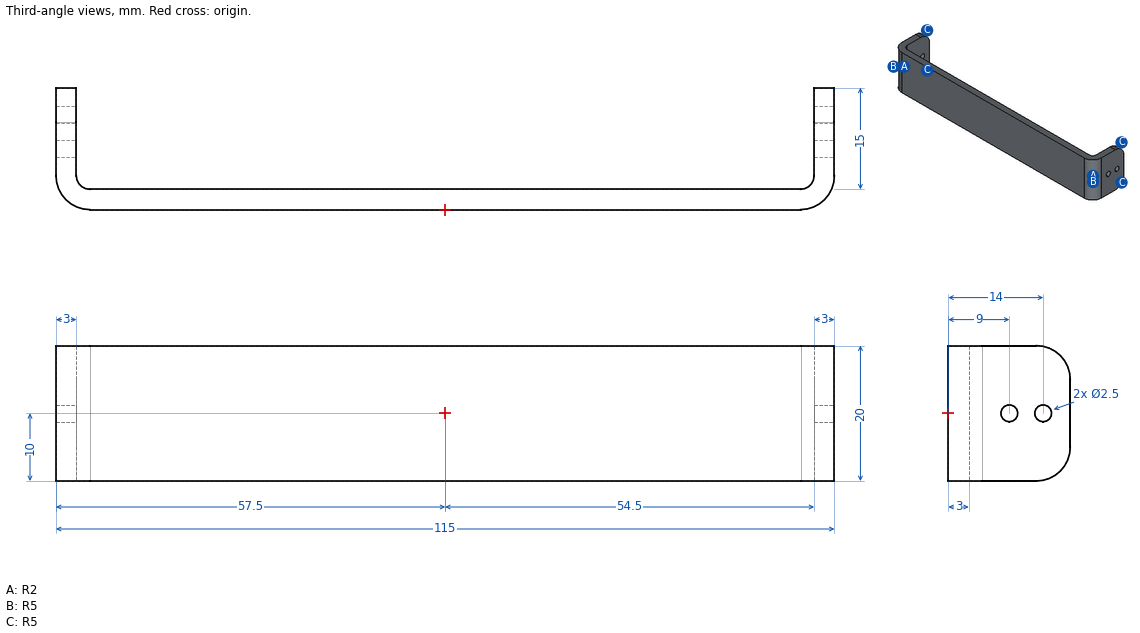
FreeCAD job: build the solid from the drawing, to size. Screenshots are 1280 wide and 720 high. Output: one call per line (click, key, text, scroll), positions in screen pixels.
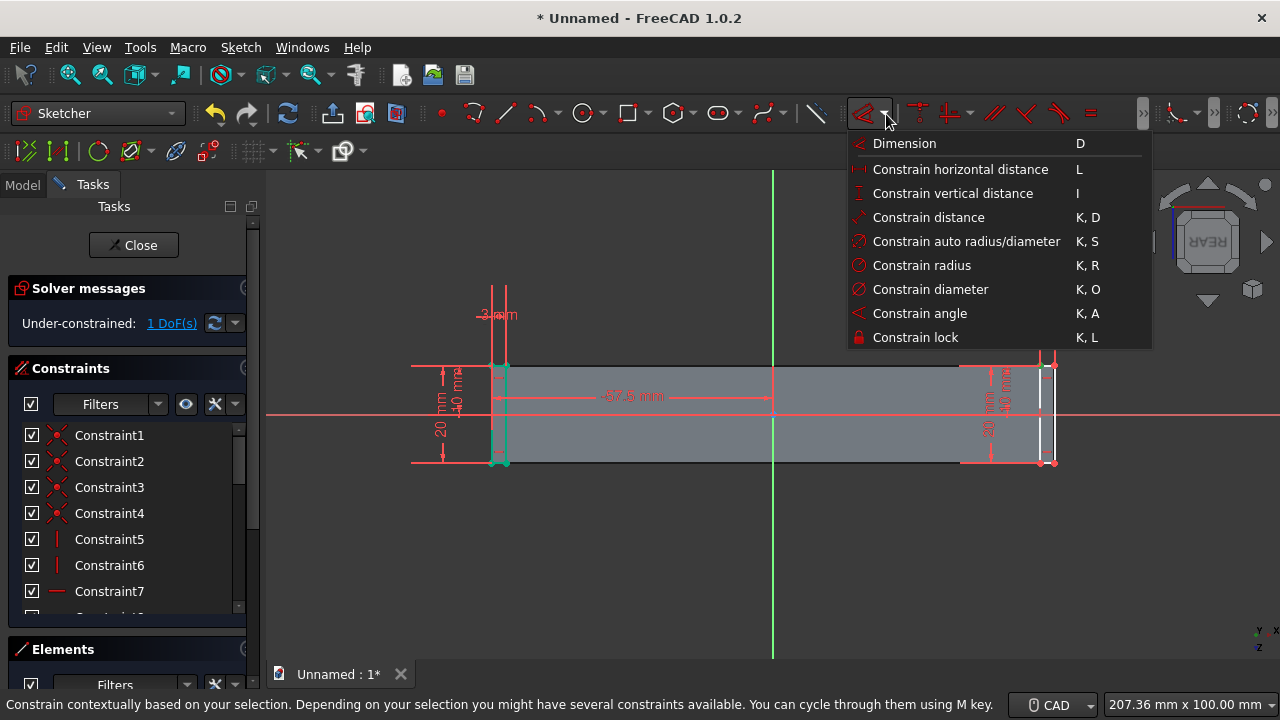
click(1000, 169)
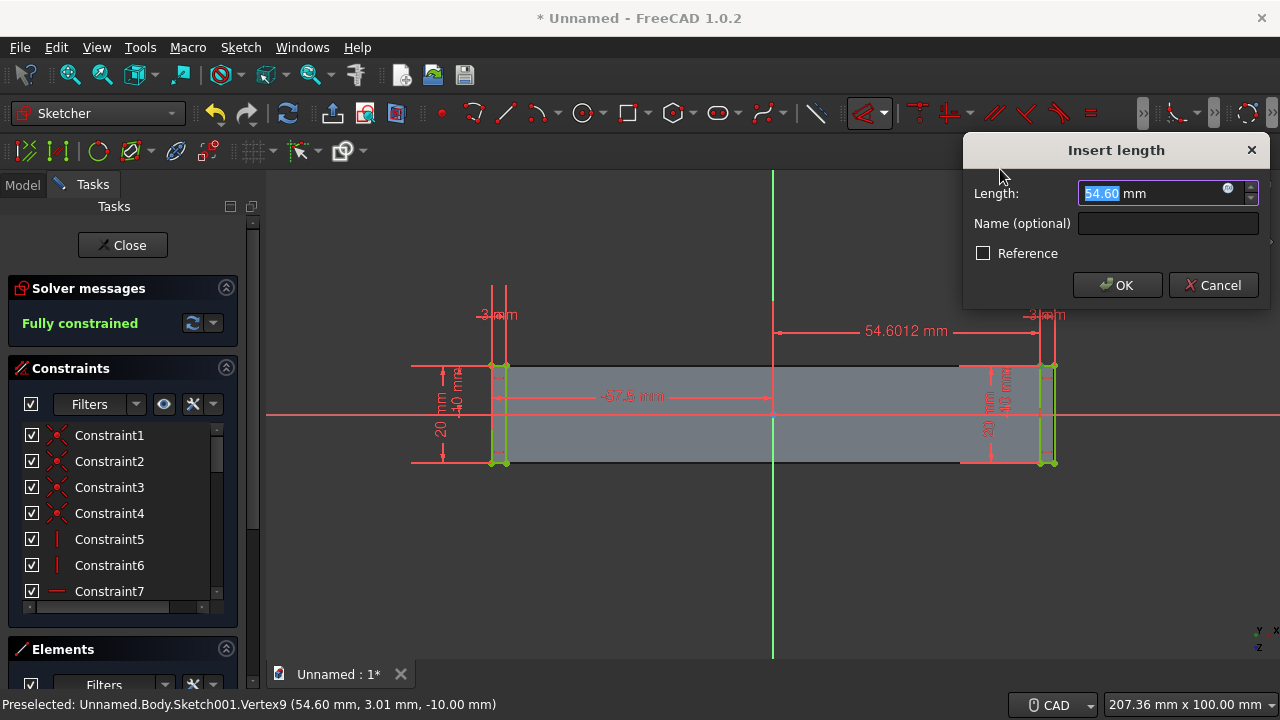
text(54.5)
key(Return)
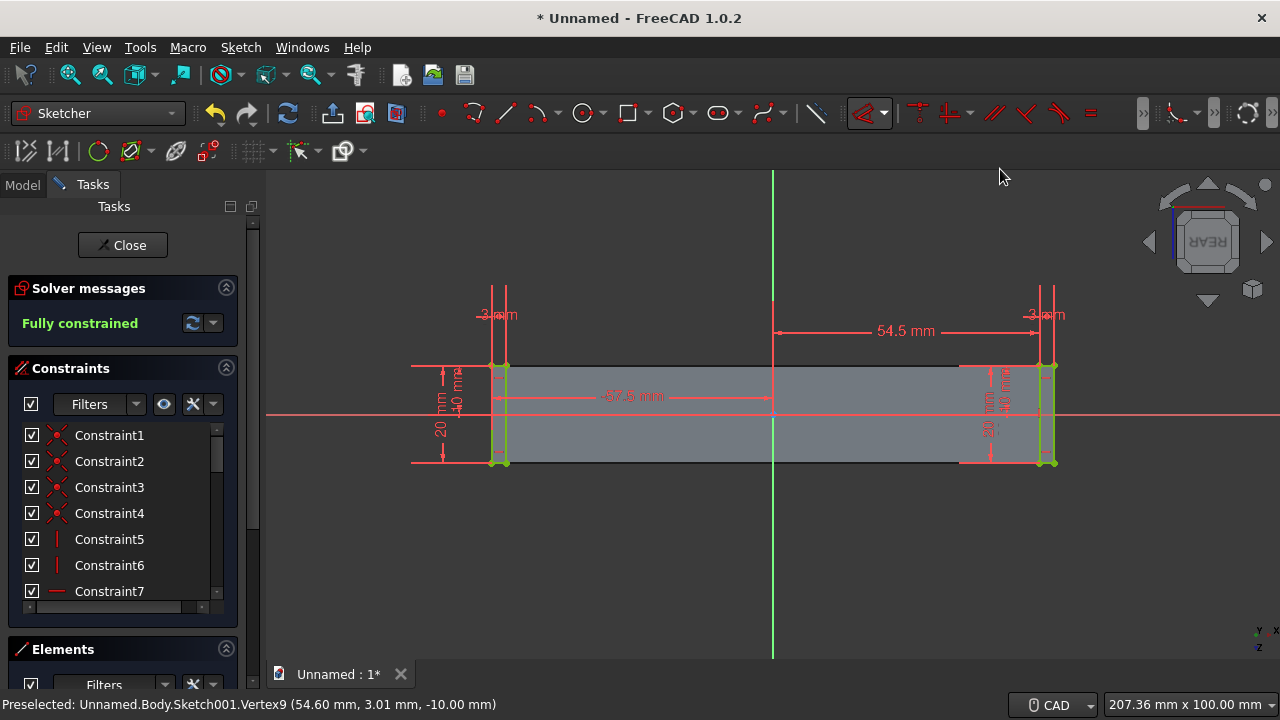
click(123, 245)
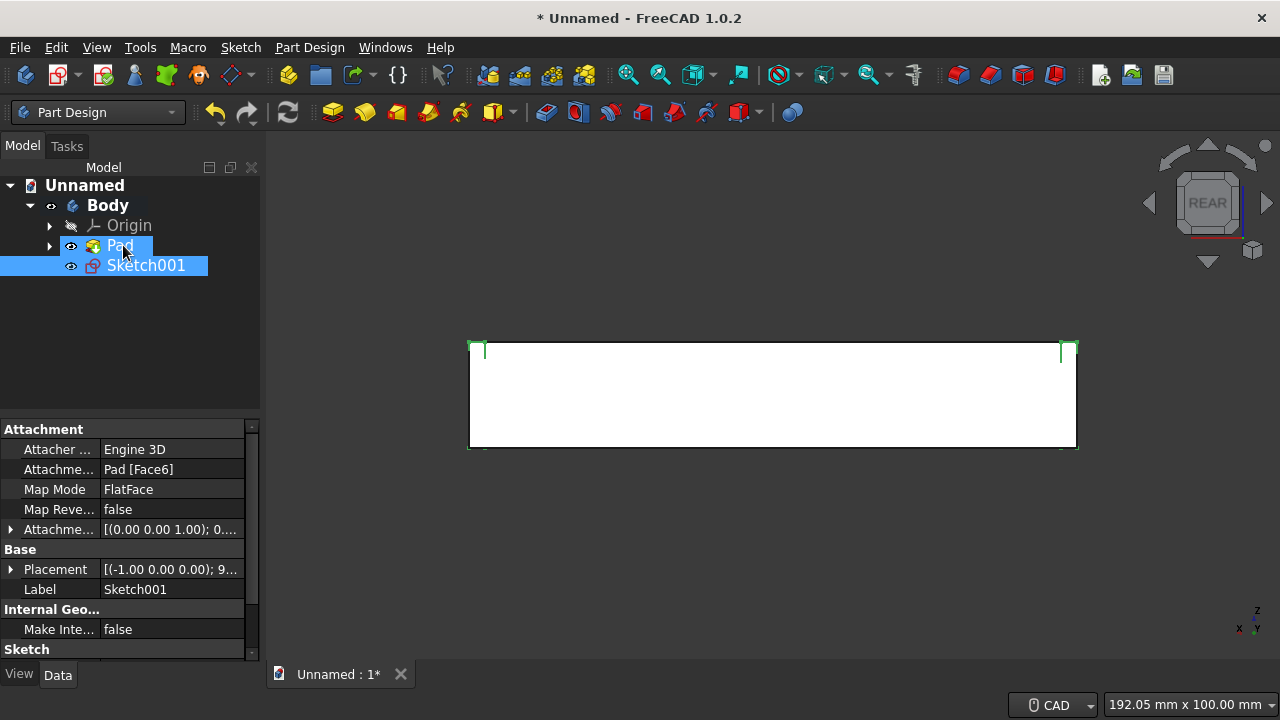
click(334, 112)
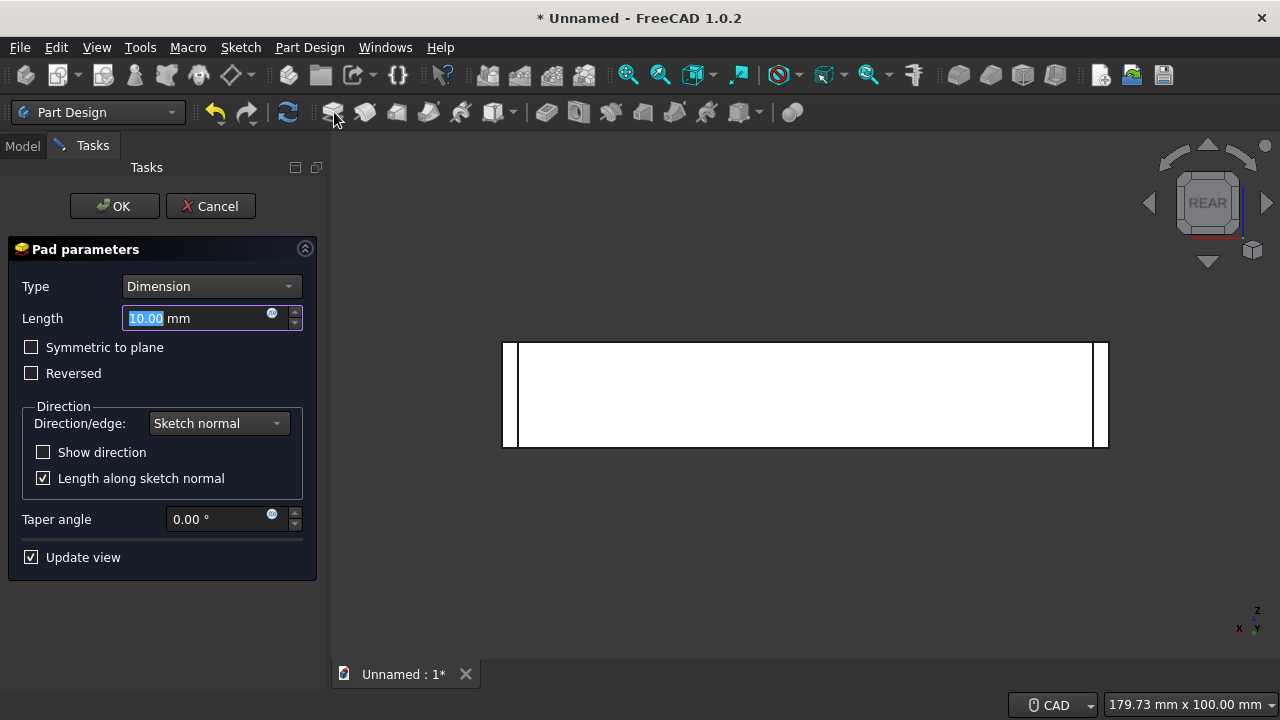
text(15)
key(Tab)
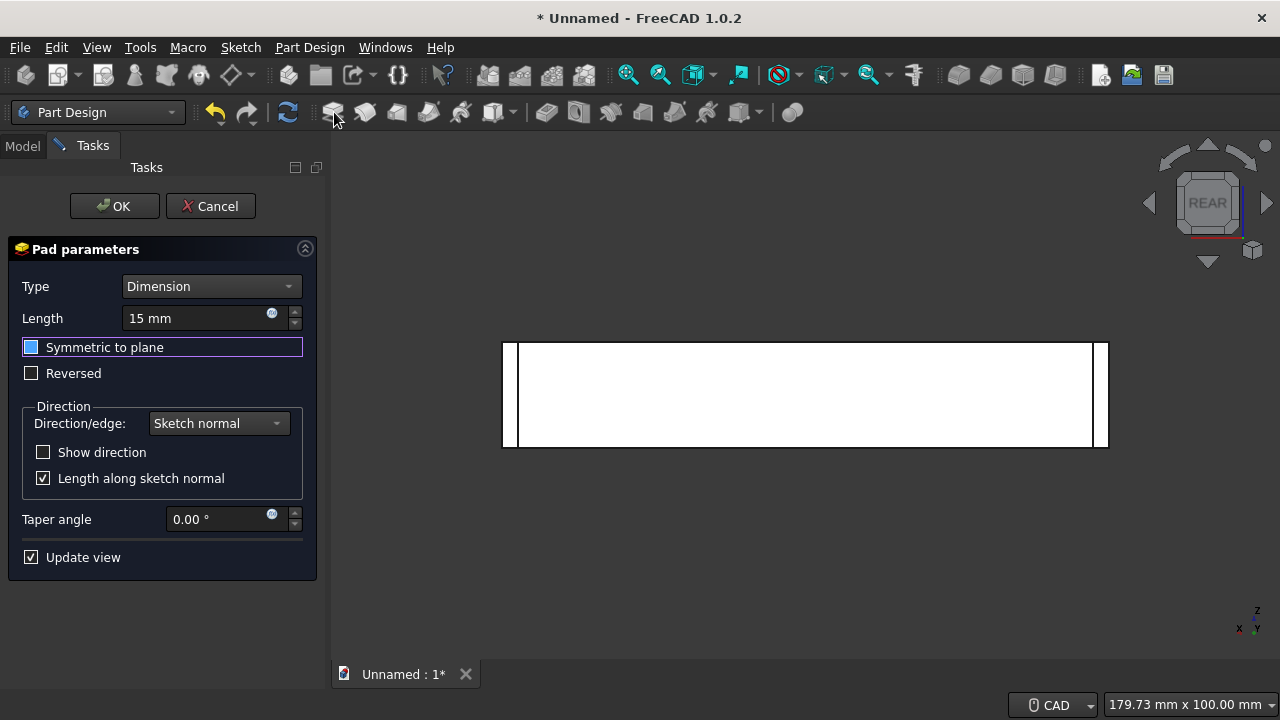
click(115, 206)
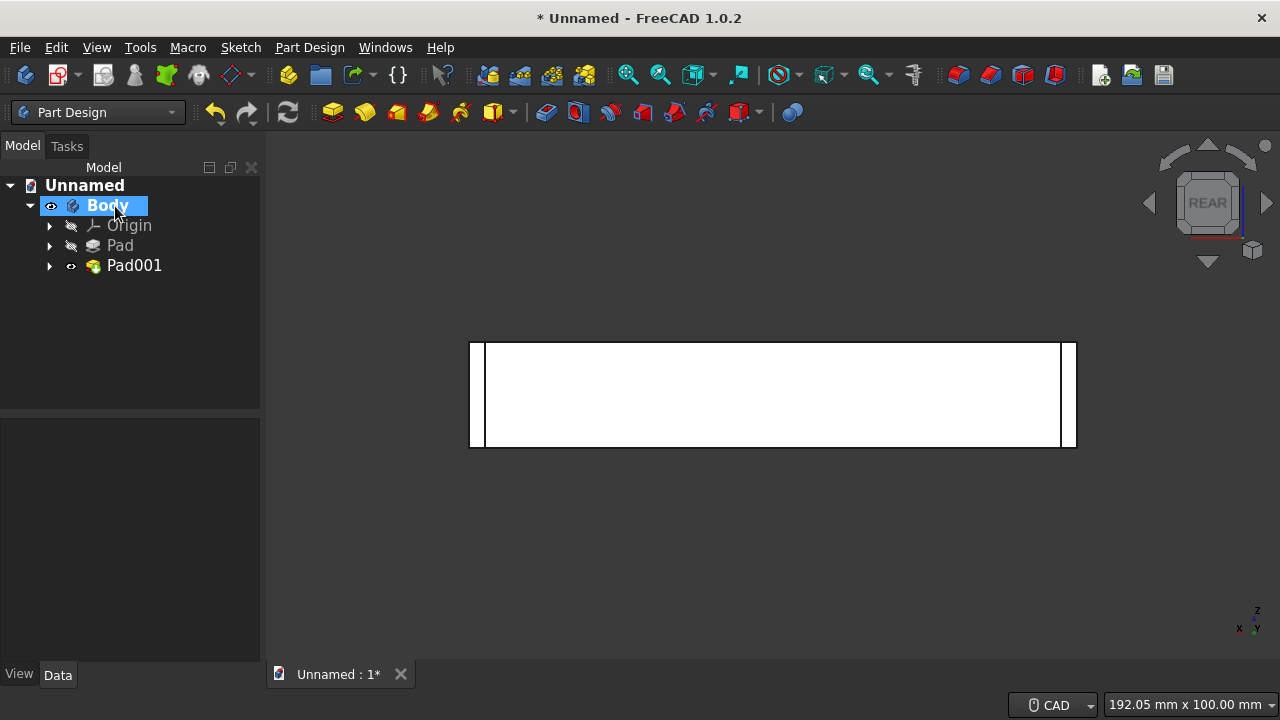
key(0)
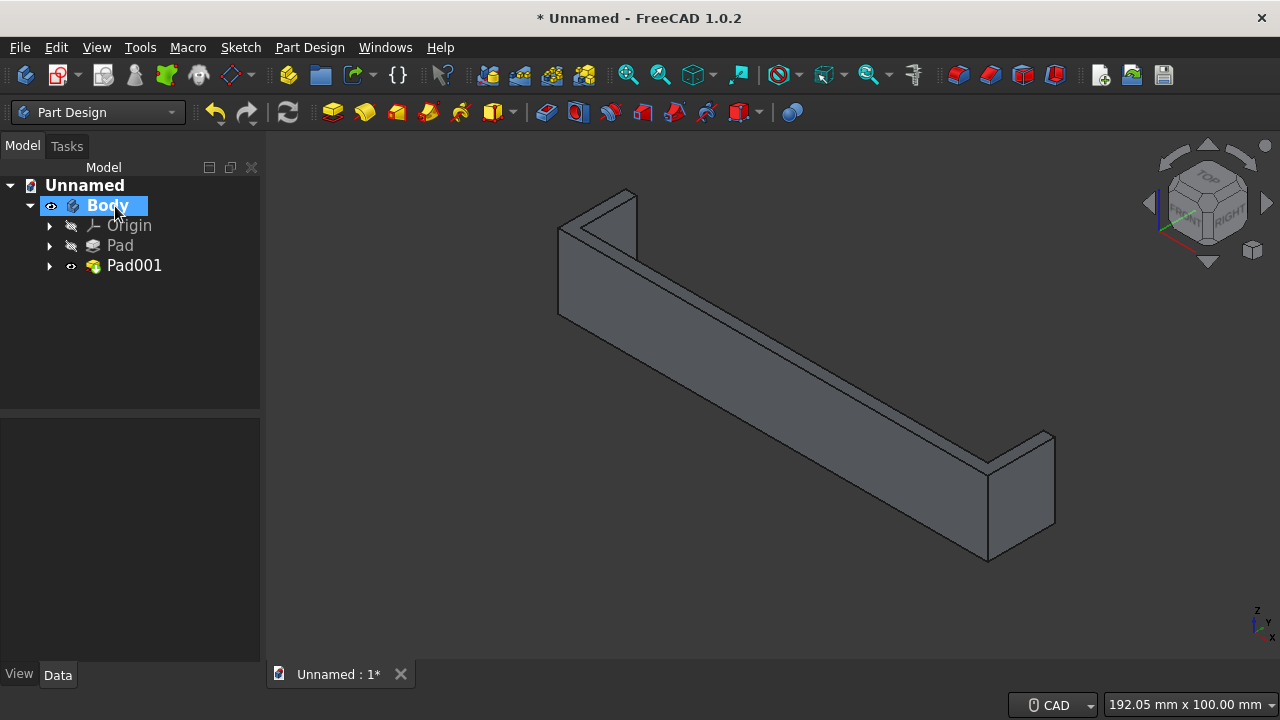
key(2)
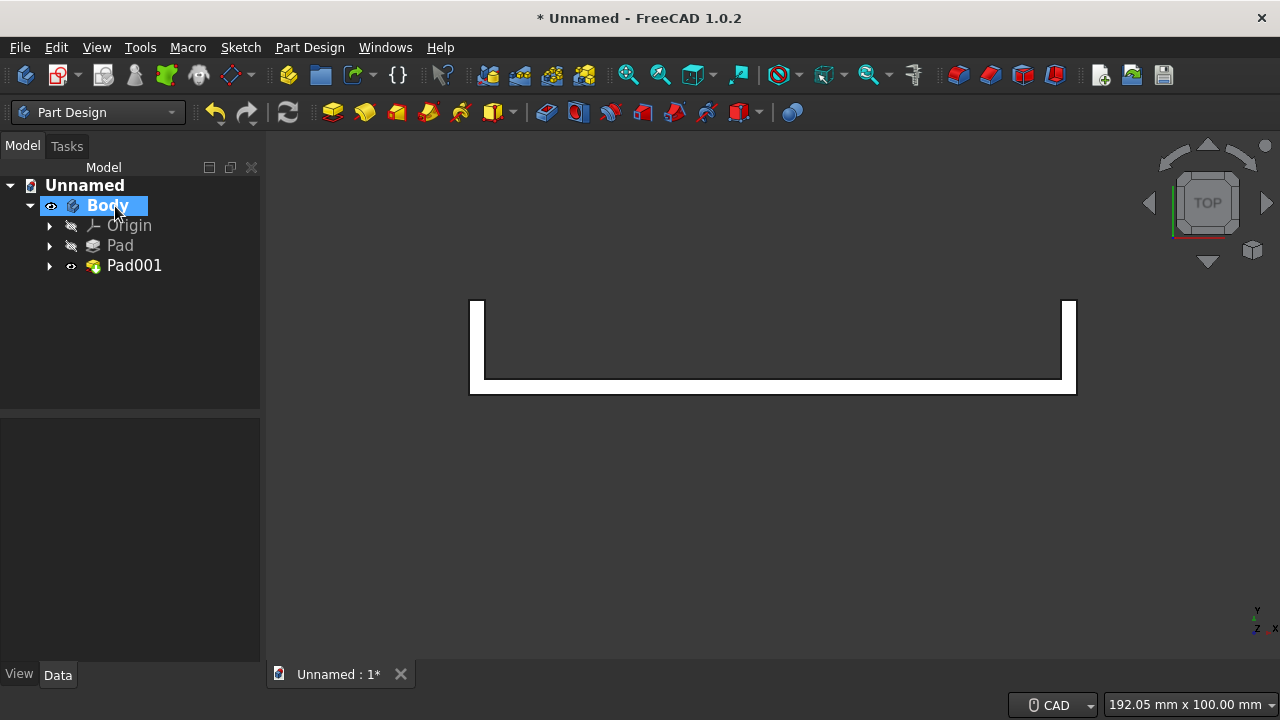
key(1)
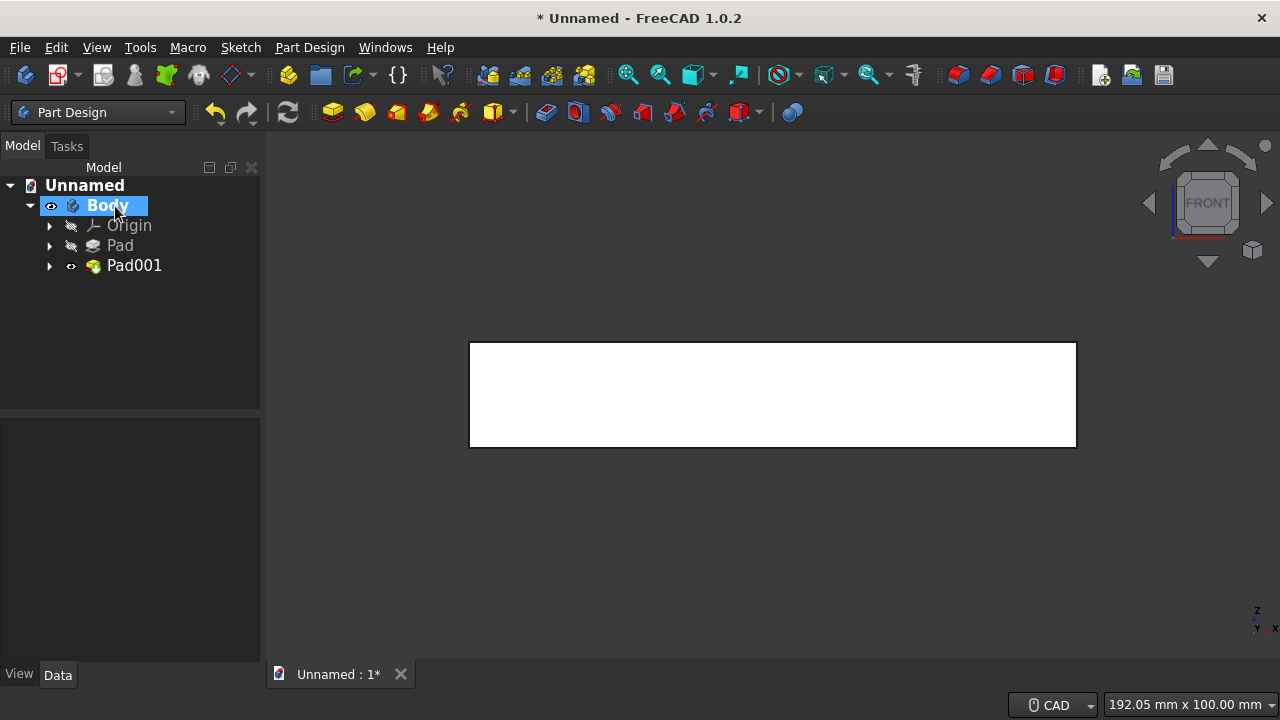
key(3)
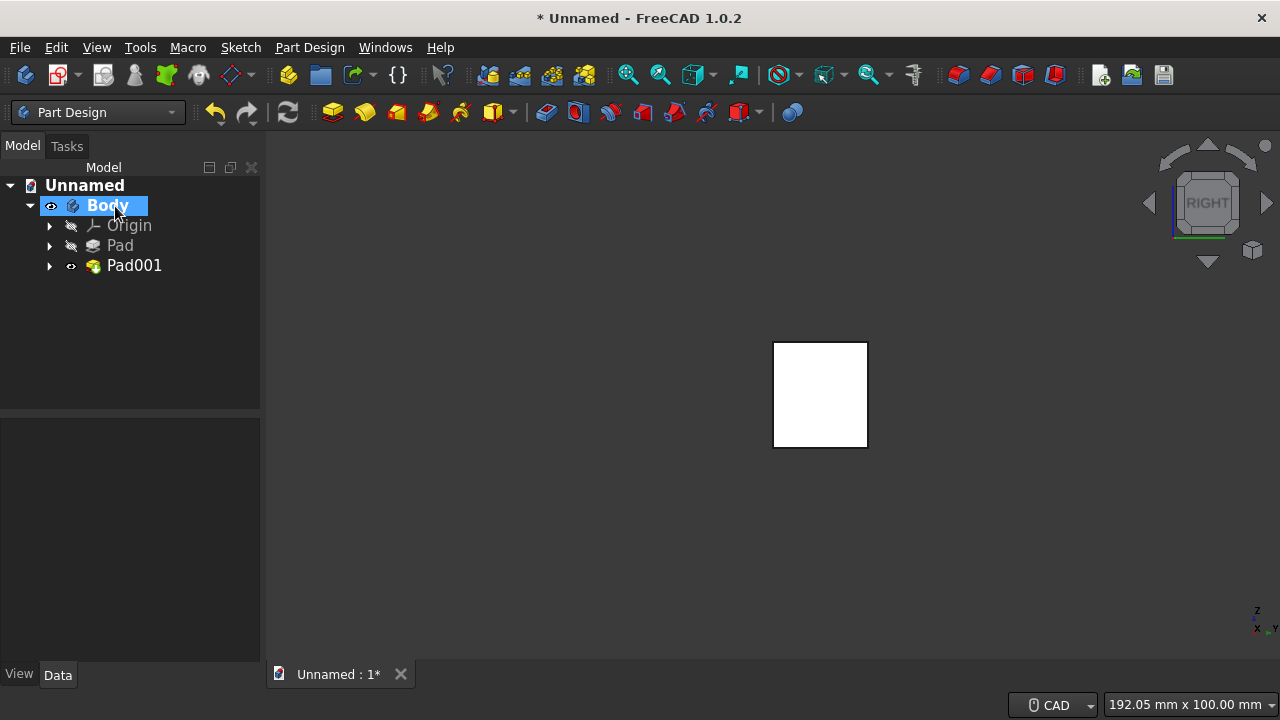
click(630, 76)